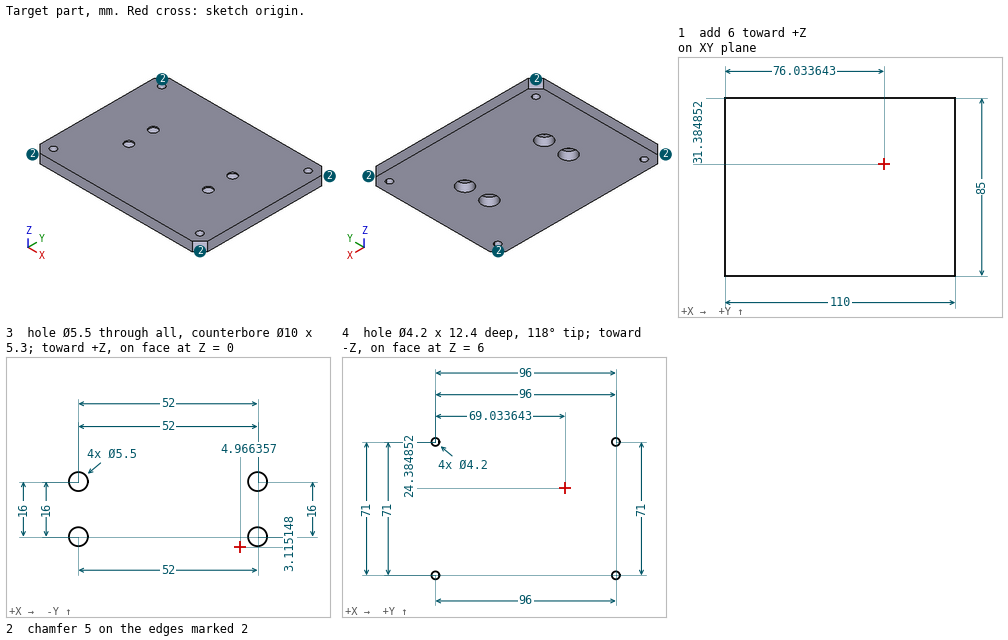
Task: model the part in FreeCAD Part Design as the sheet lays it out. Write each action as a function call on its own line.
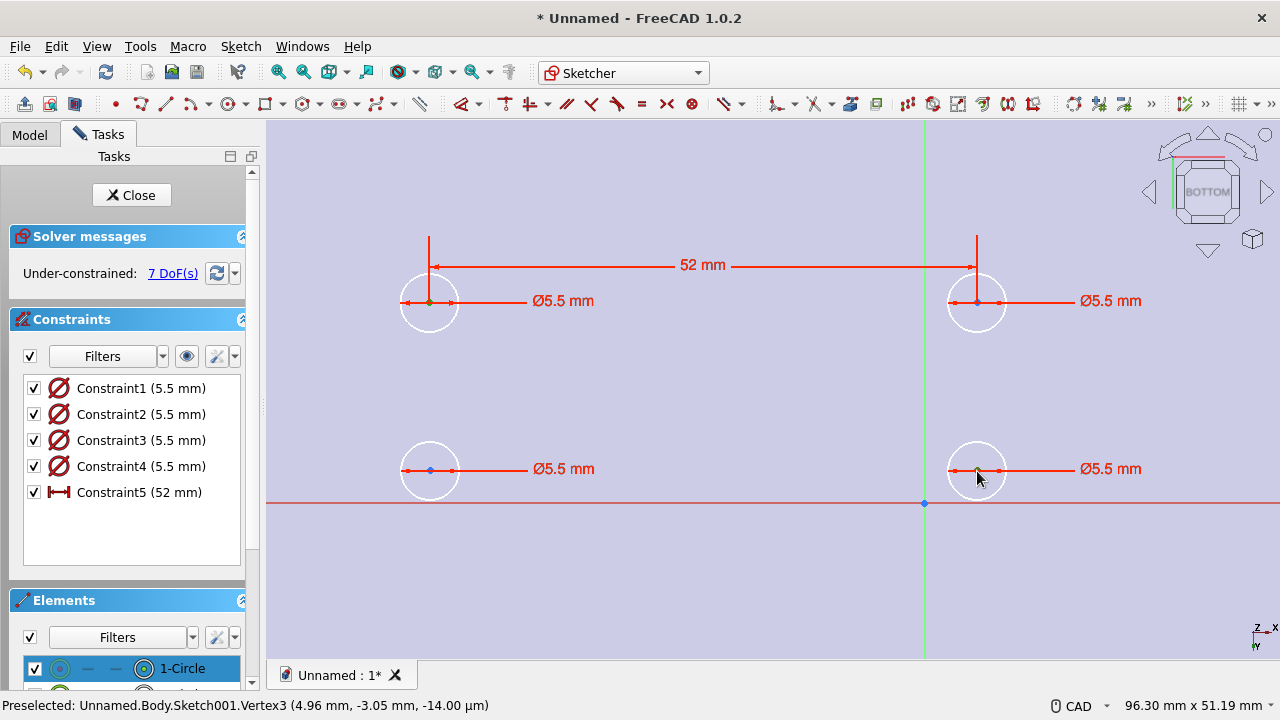
key(l)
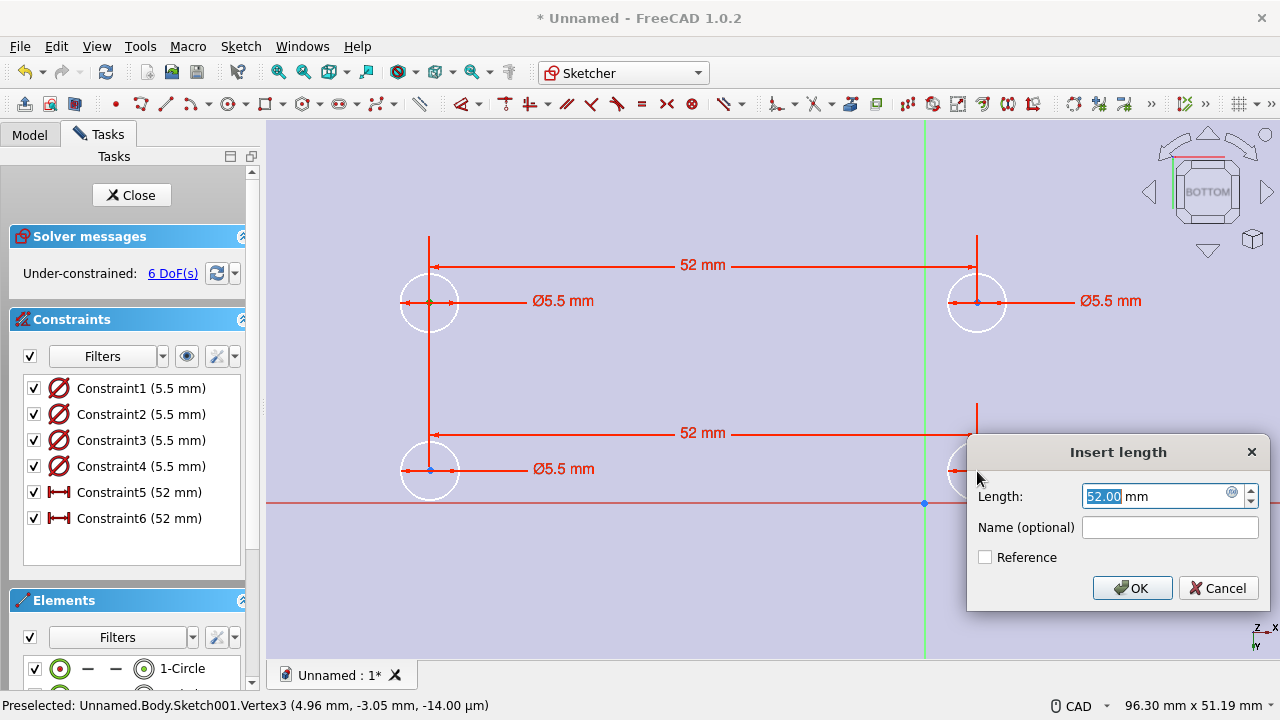
text(52)
key(Return)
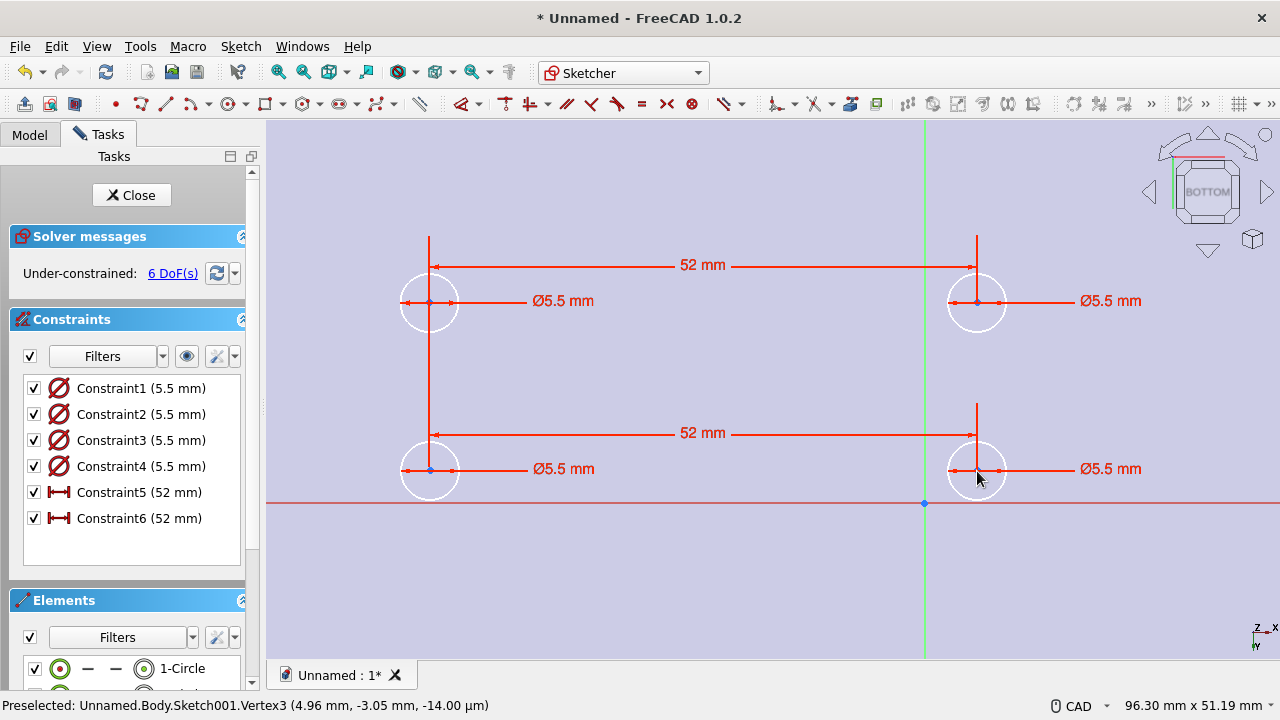
click(977, 303)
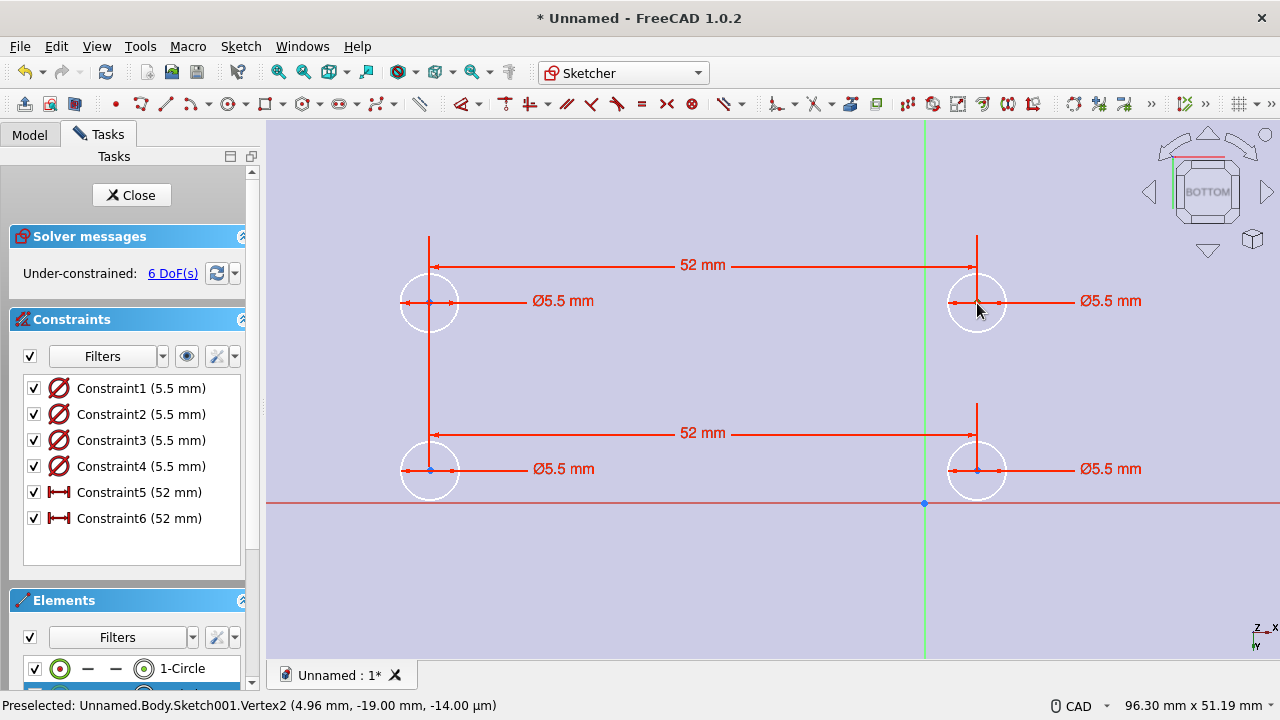
click(977, 471)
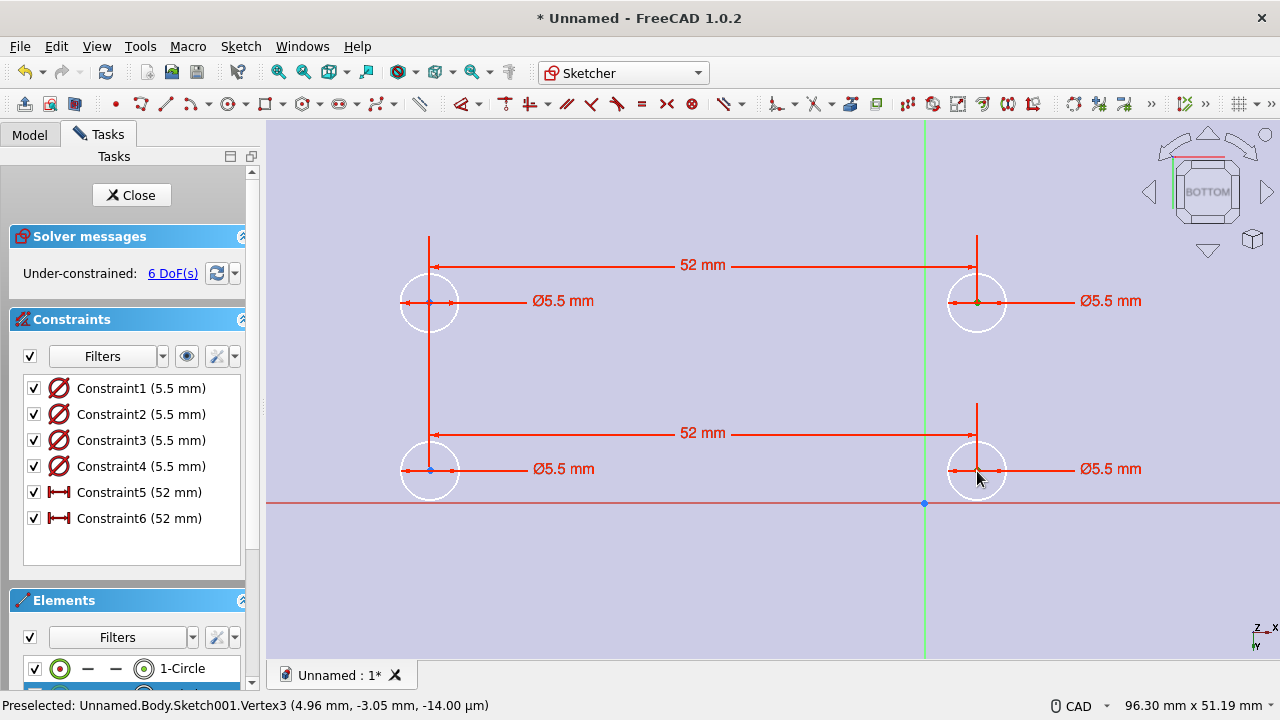
key(i)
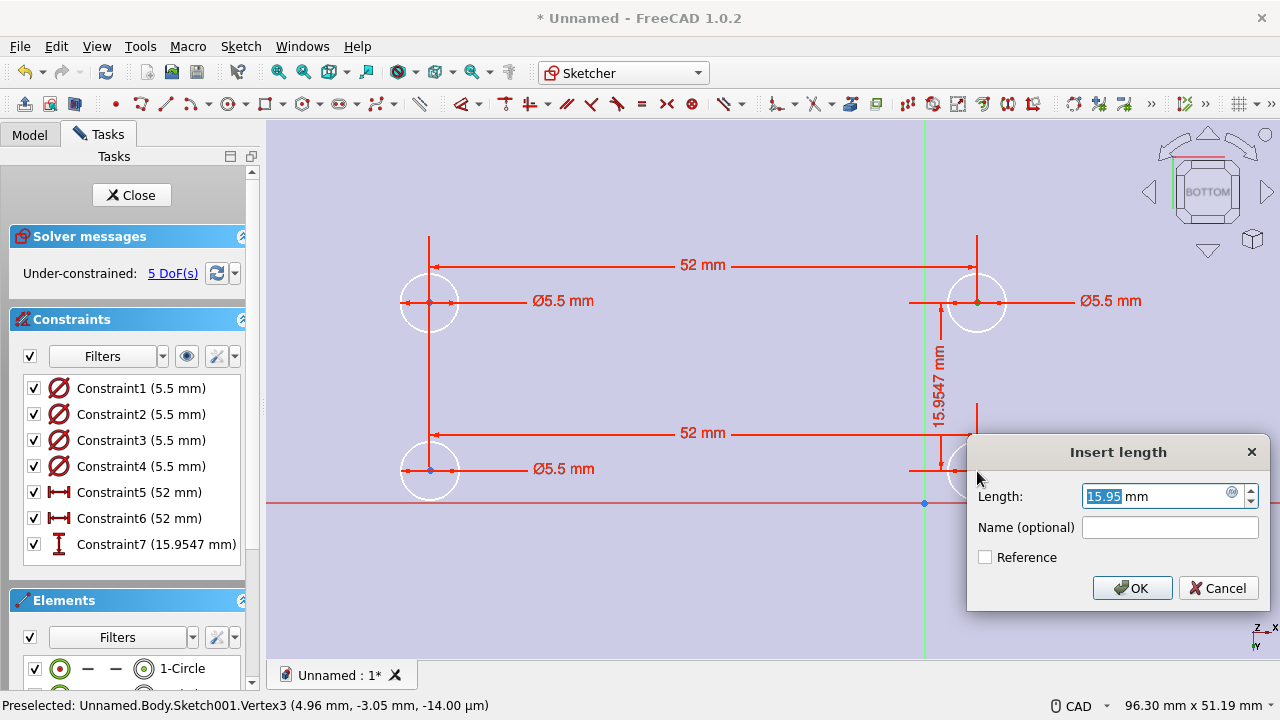
text(16)
key(Return)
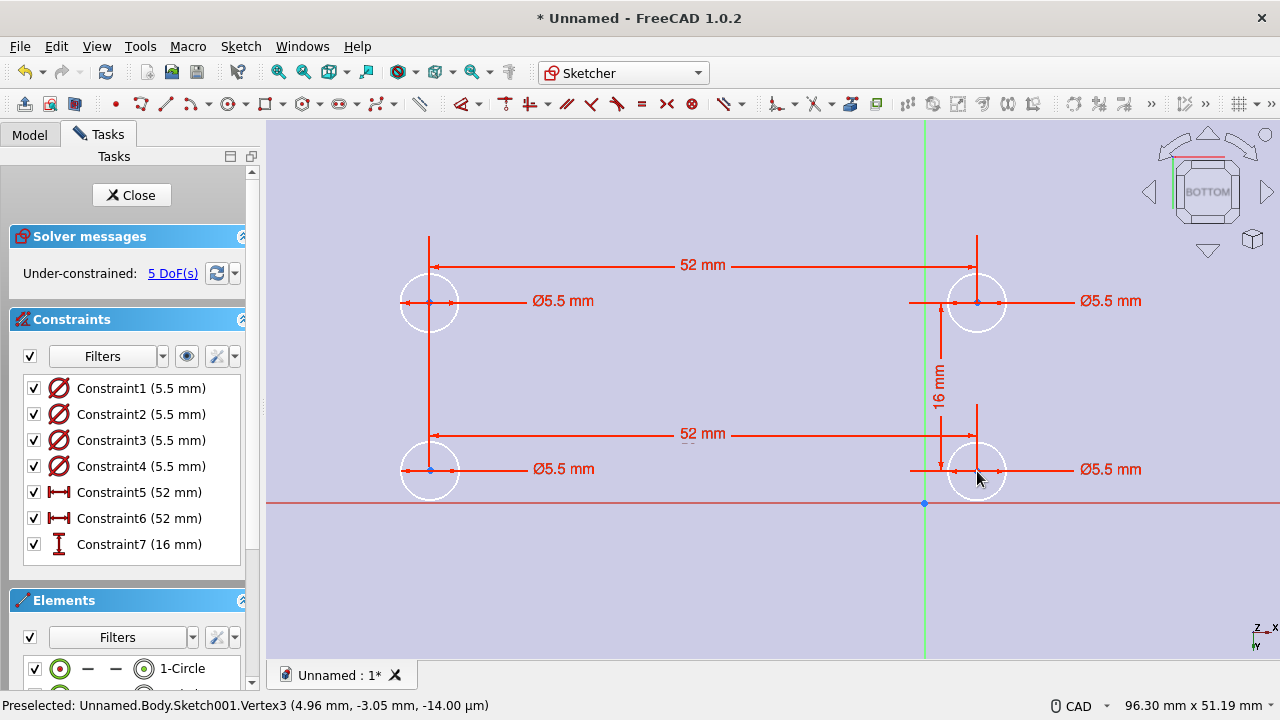
click(429, 303)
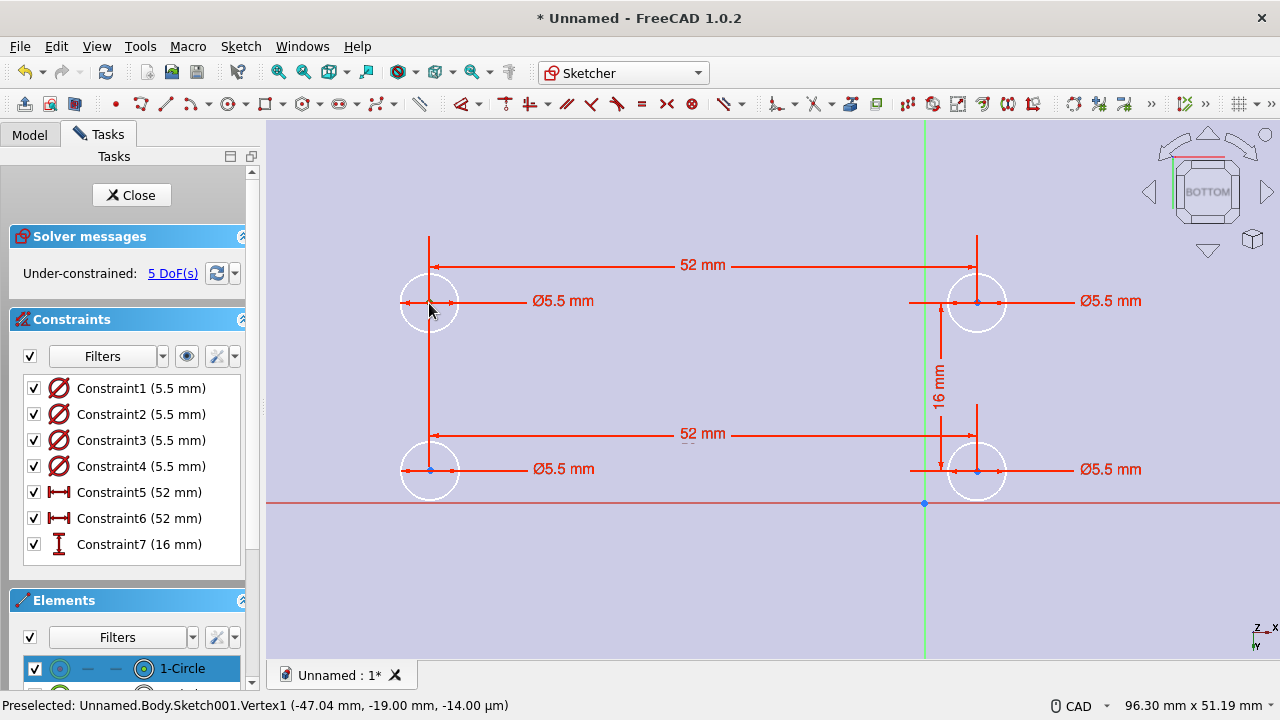
click(977, 471)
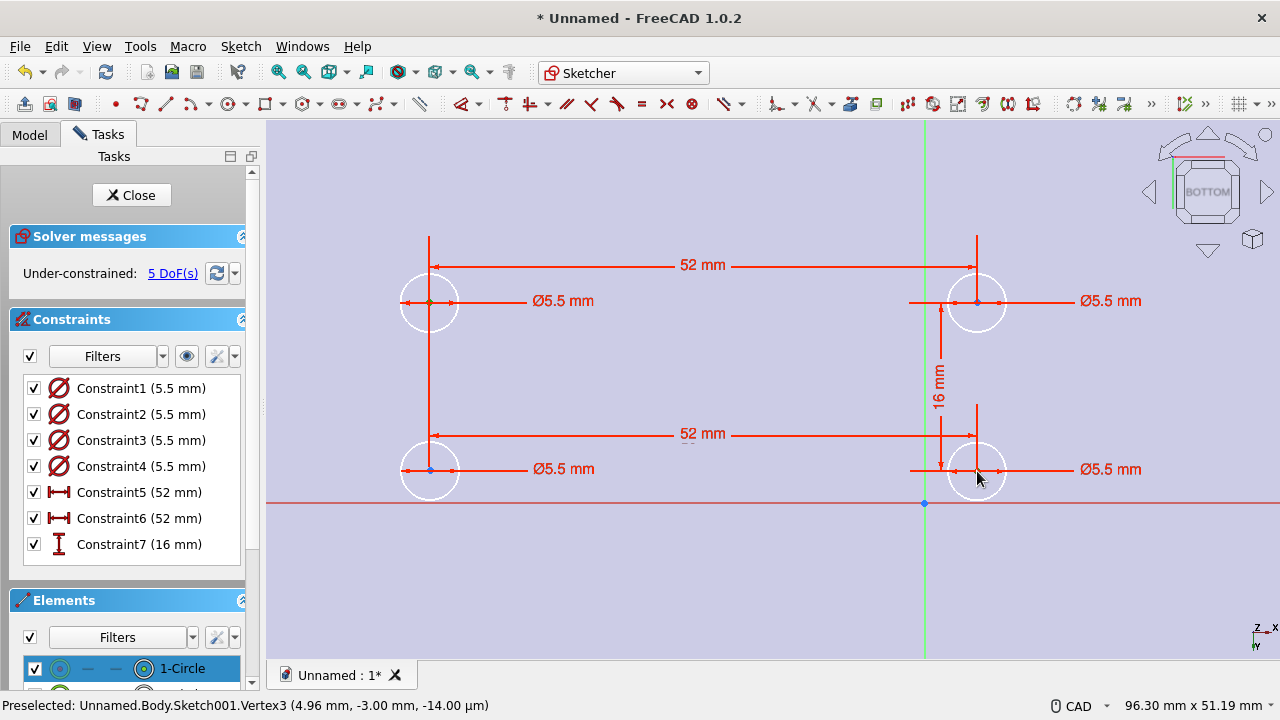
key(i)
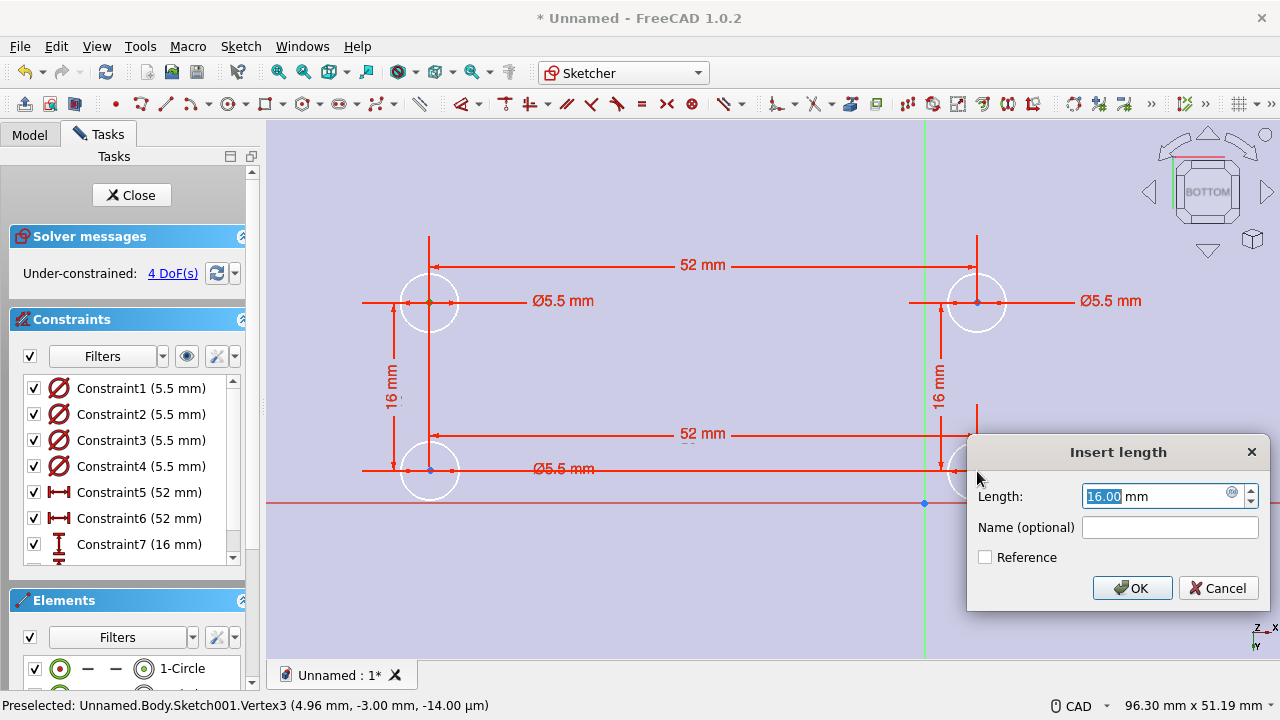
text(16)
key(Return)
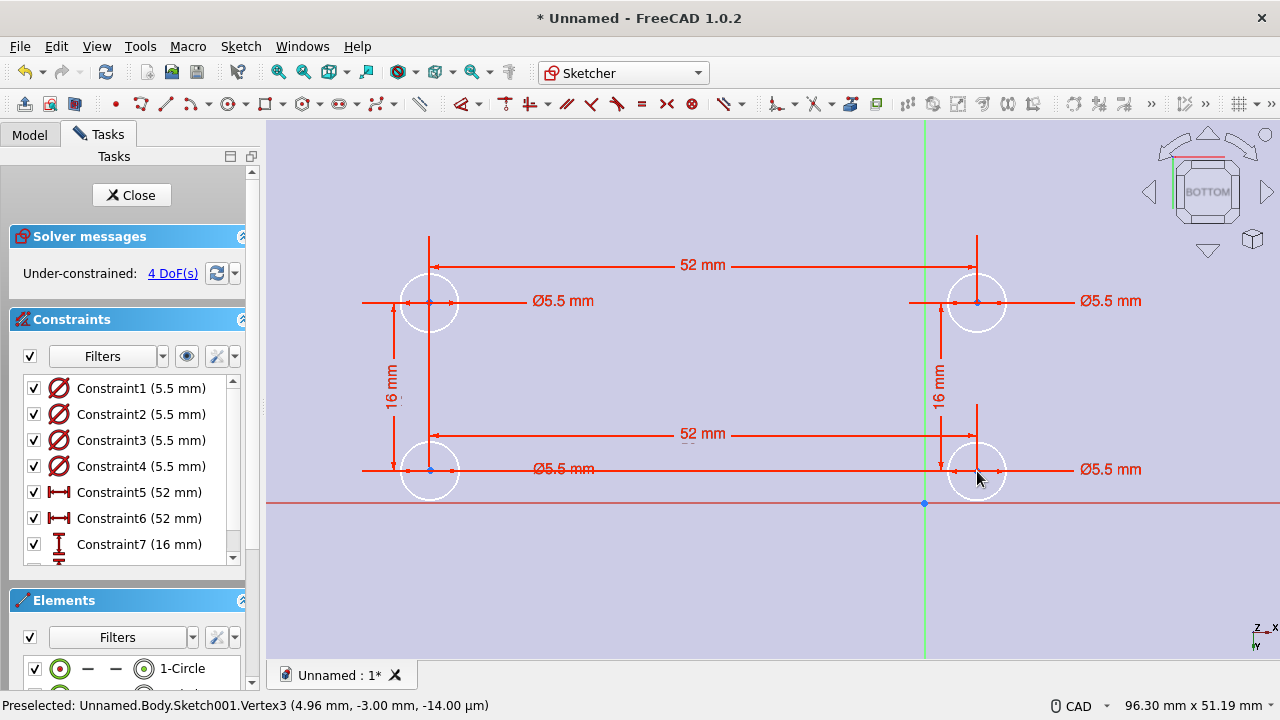
click(977, 471)